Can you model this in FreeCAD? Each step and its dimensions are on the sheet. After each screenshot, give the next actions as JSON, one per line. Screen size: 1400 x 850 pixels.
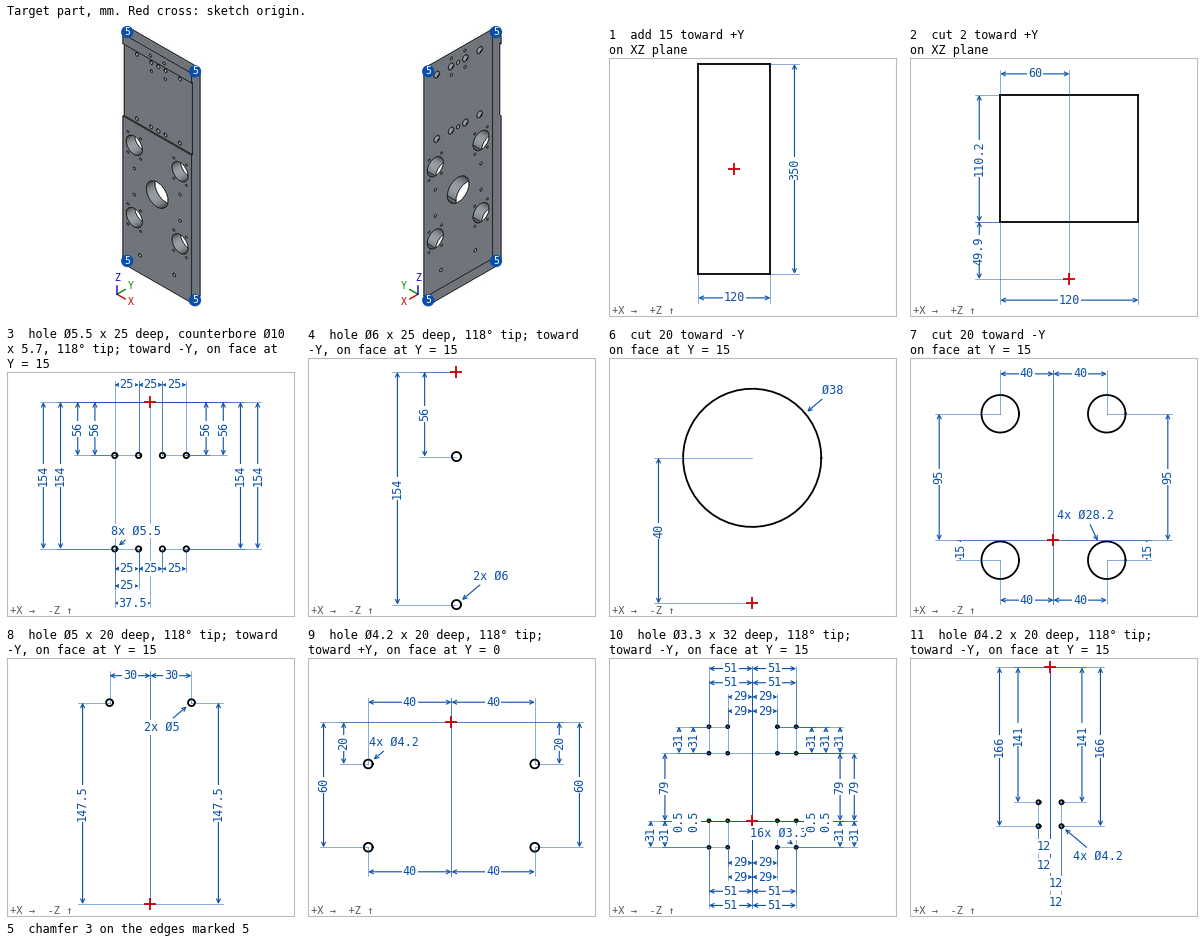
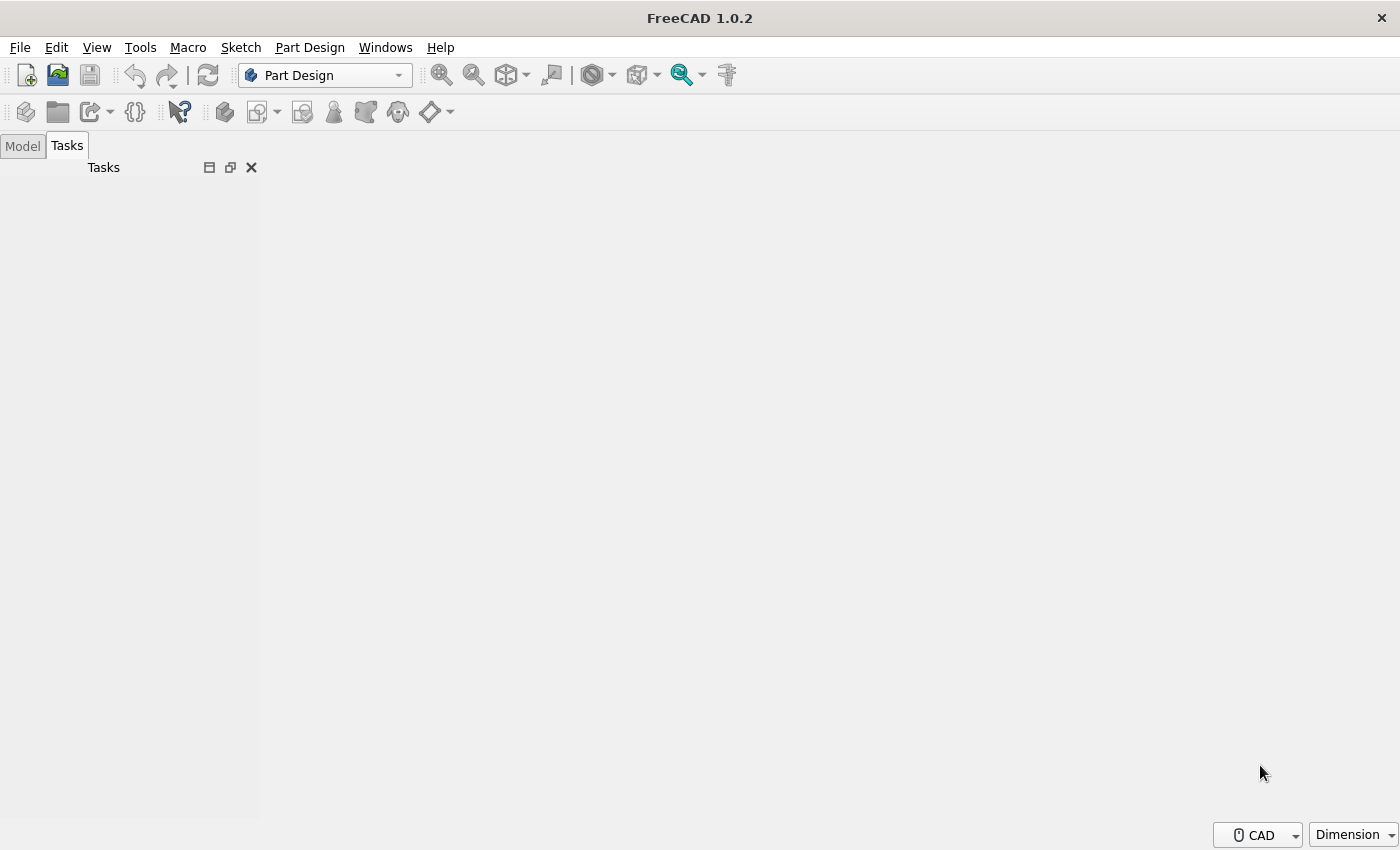
{"action": "left_click", "coordinate": [750, 112]}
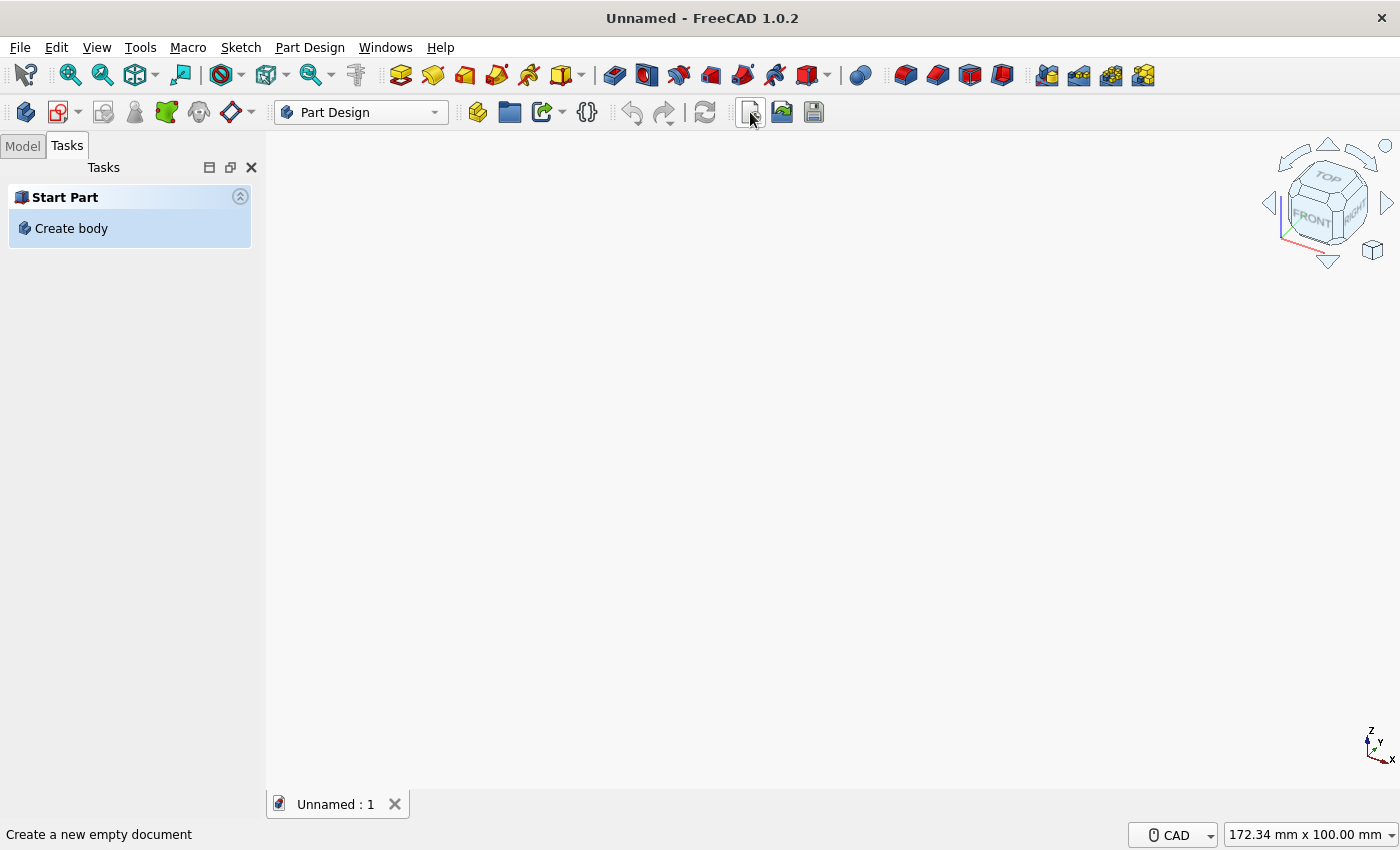
{"action": "left_click", "coordinate": [58, 112]}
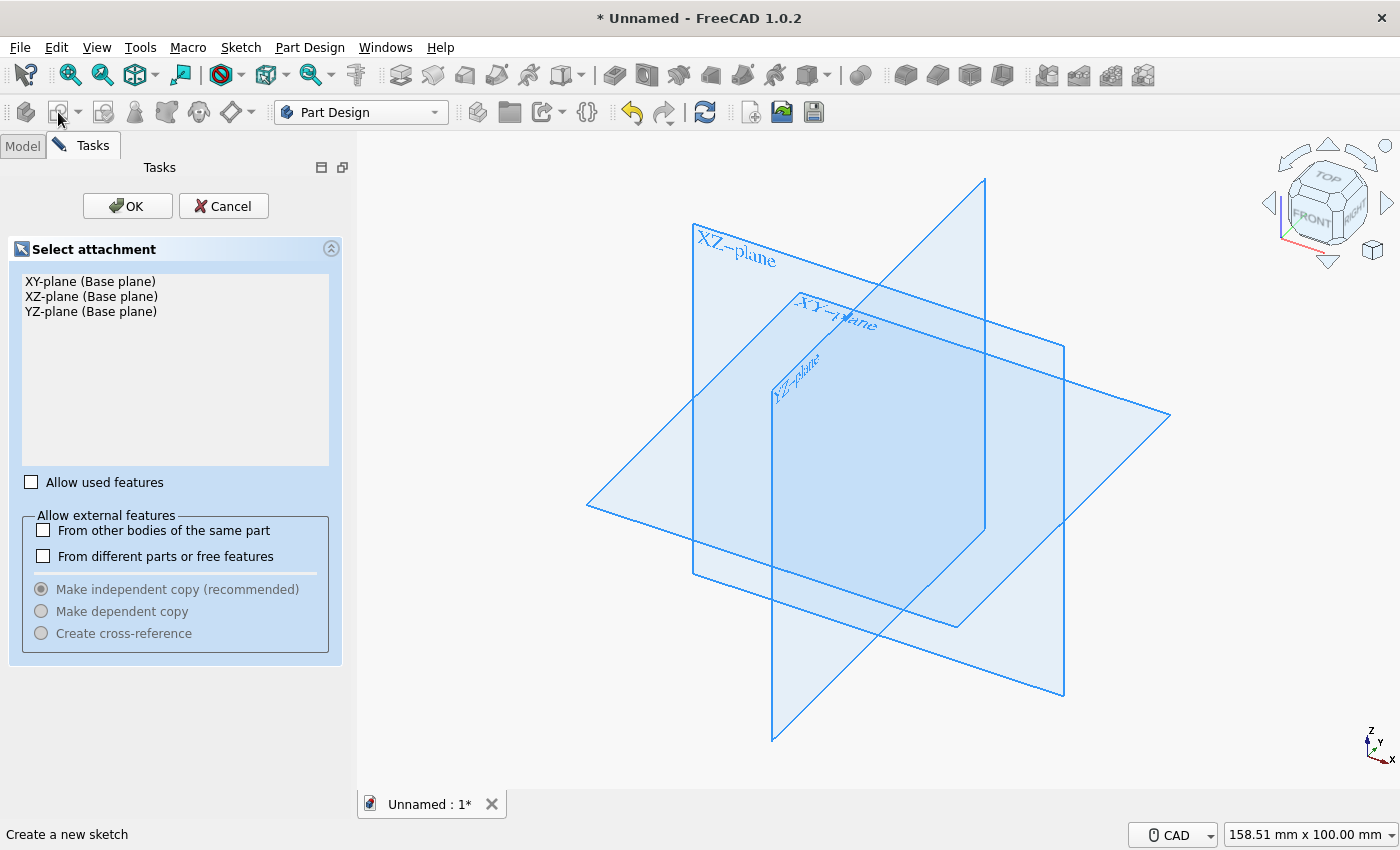
{"action": "left_click", "coordinate": [82, 296]}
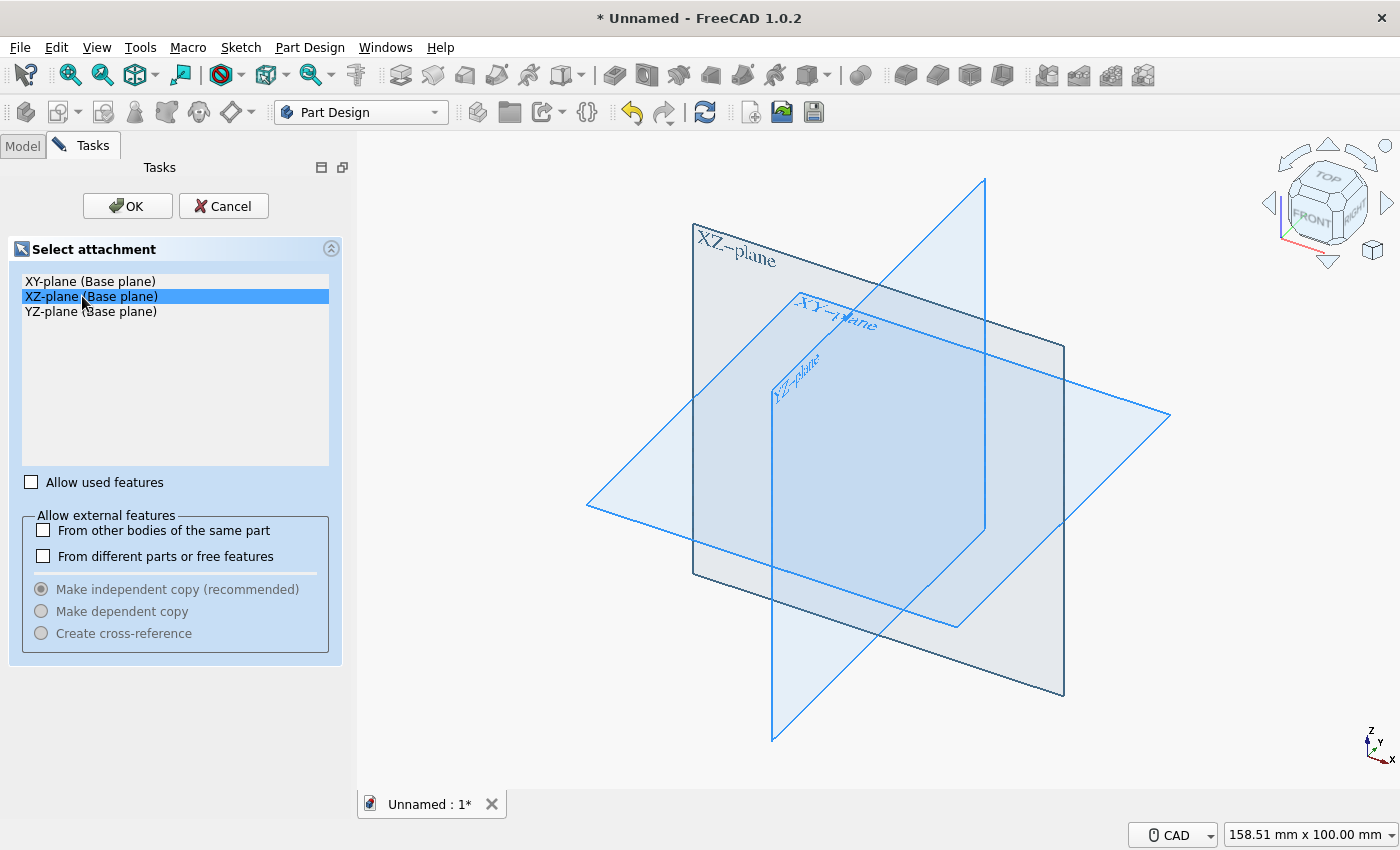
{"action": "left_click", "coordinate": [128, 206]}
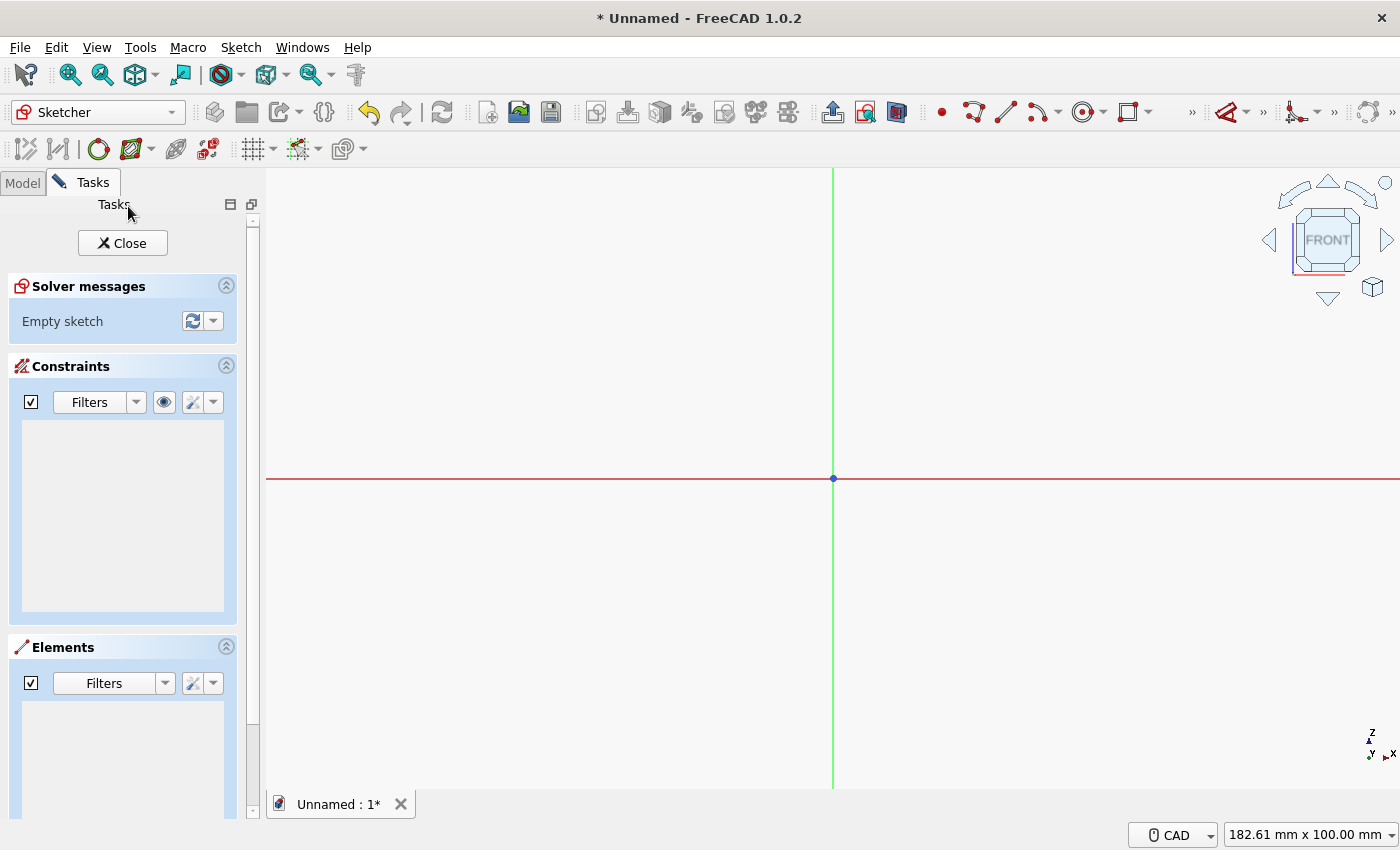
{"action": "scroll", "coordinate": [747, 478], "scroll_direction": "down", "scroll_amount": 8}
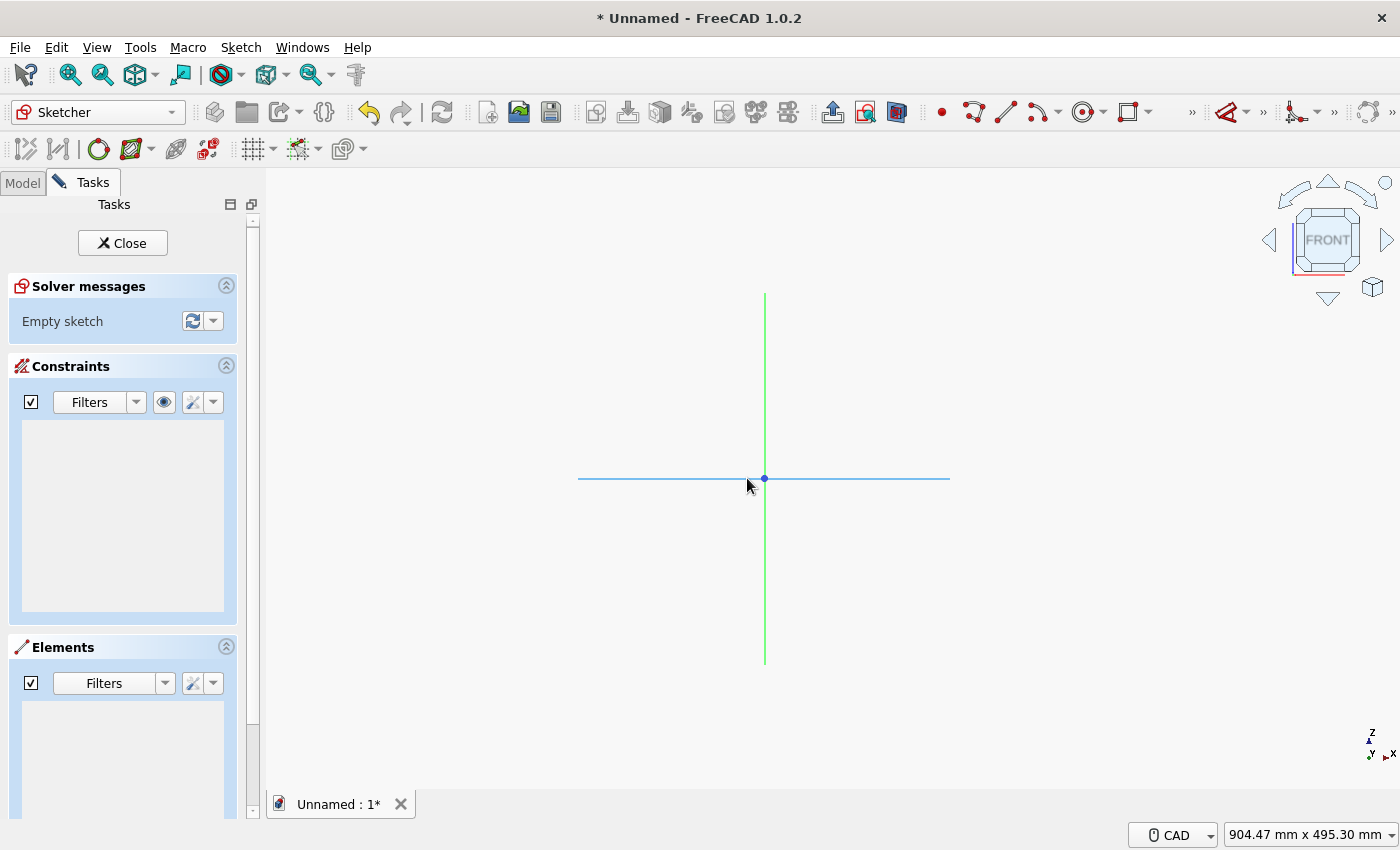
{"action": "key", "text": "g v"}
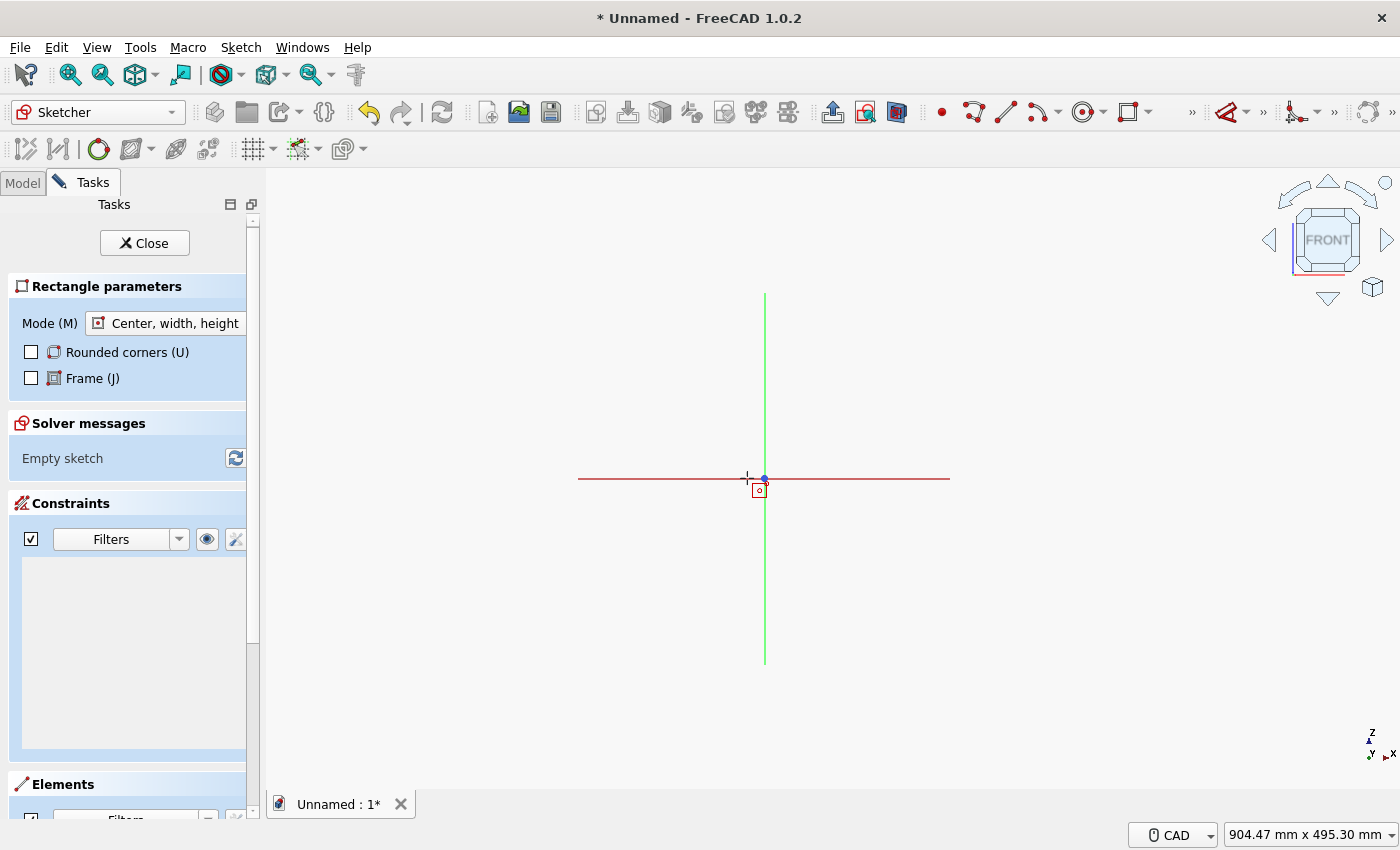
{"action": "left_click", "coordinate": [765, 478]}
{"action": "left_click", "coordinate": [840, 259]}
{"action": "key", "text": "Escape"}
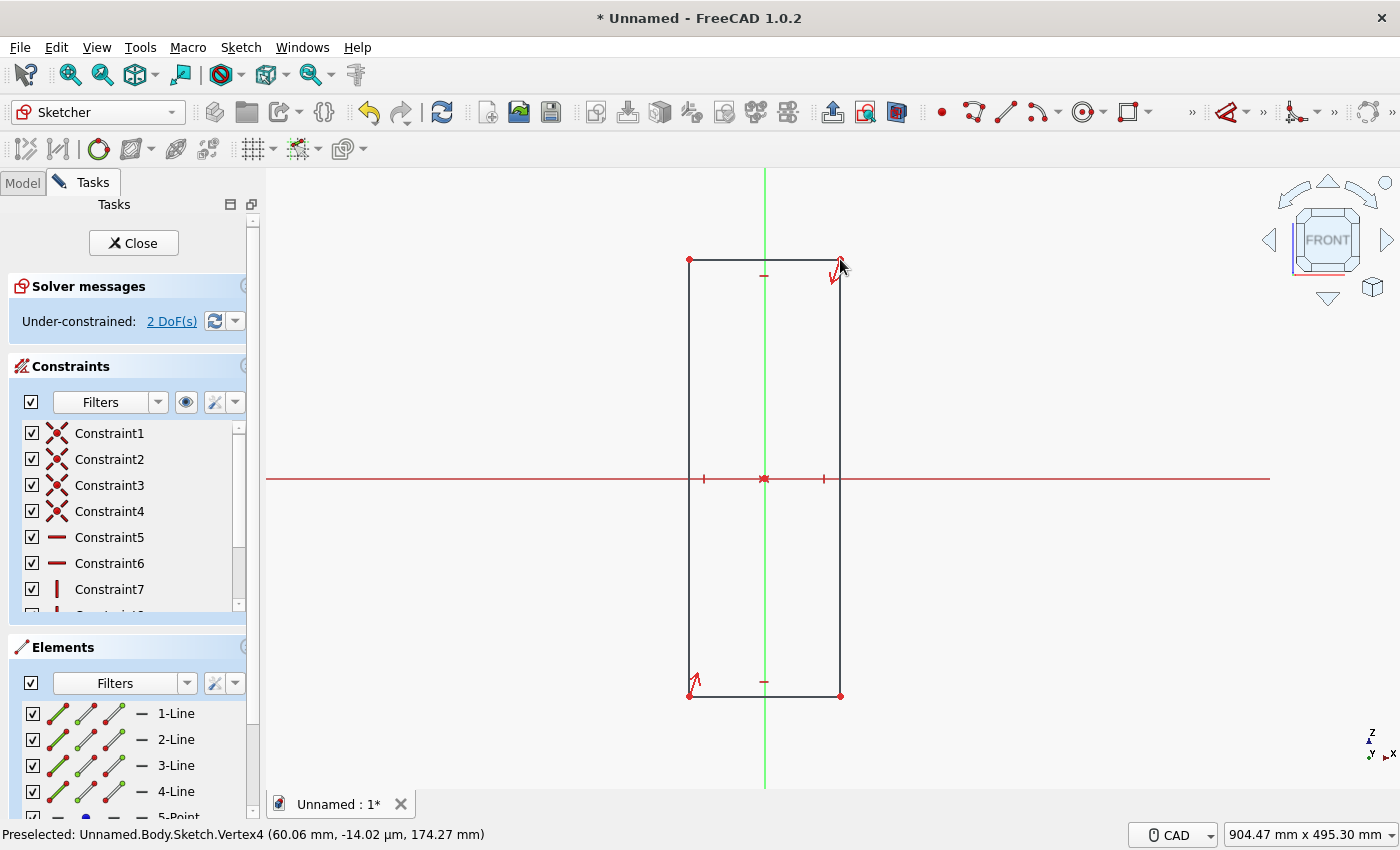
{"action": "left_click", "coordinate": [1226, 112]}